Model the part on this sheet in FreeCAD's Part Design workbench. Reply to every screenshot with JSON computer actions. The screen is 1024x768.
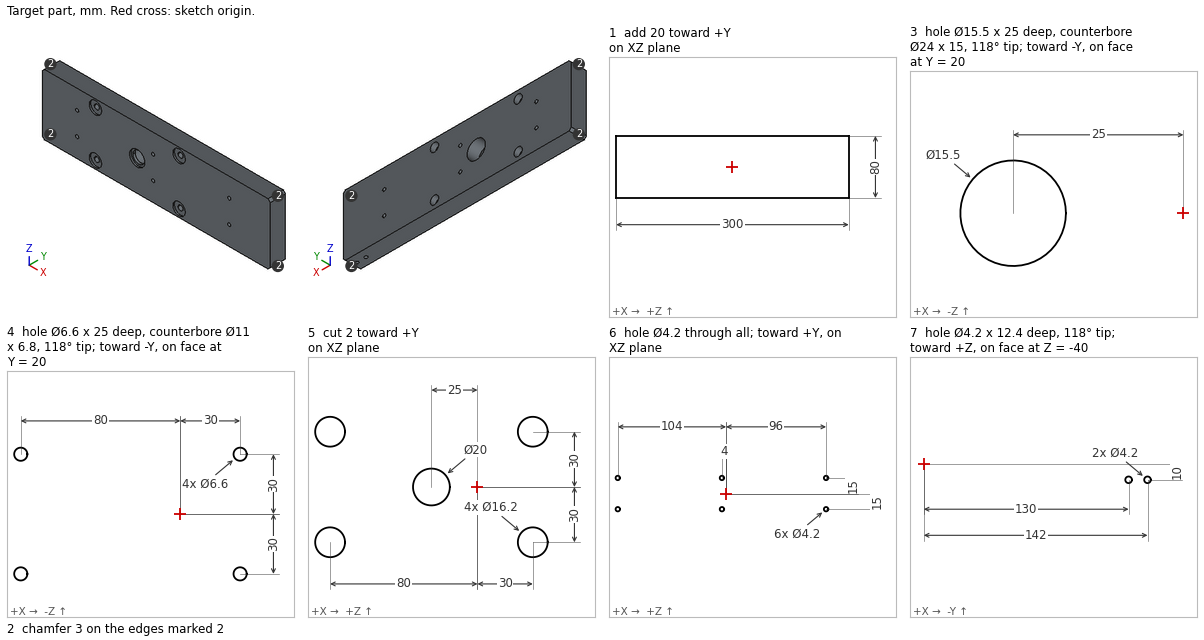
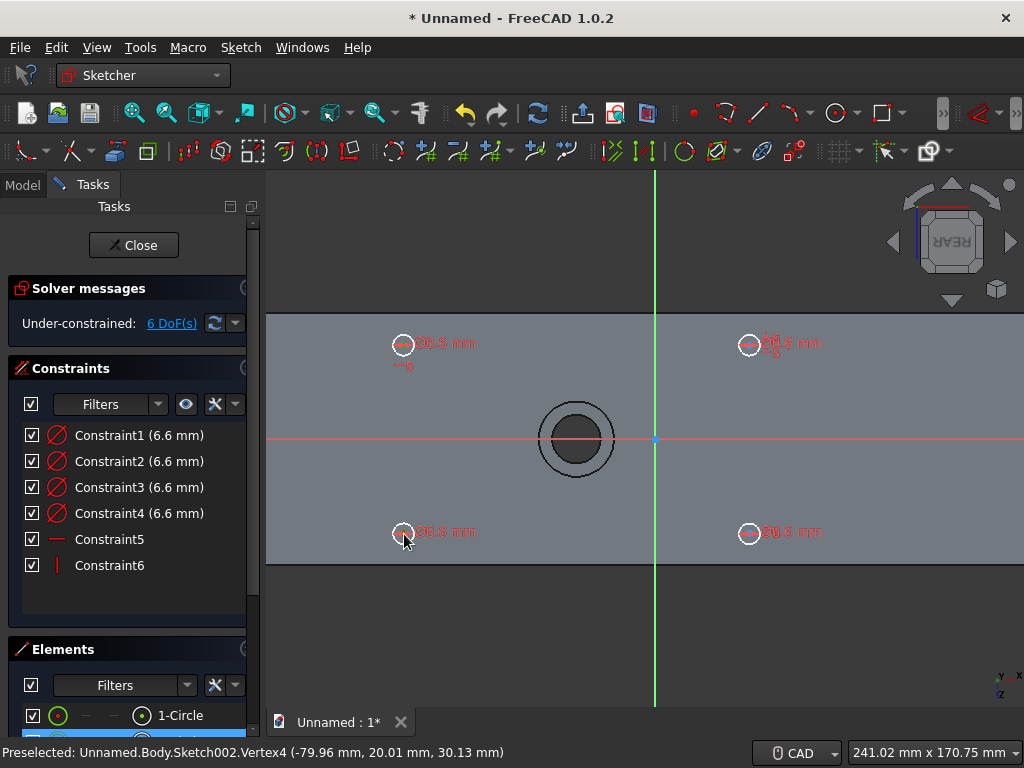
{"action": "key", "text": "v"}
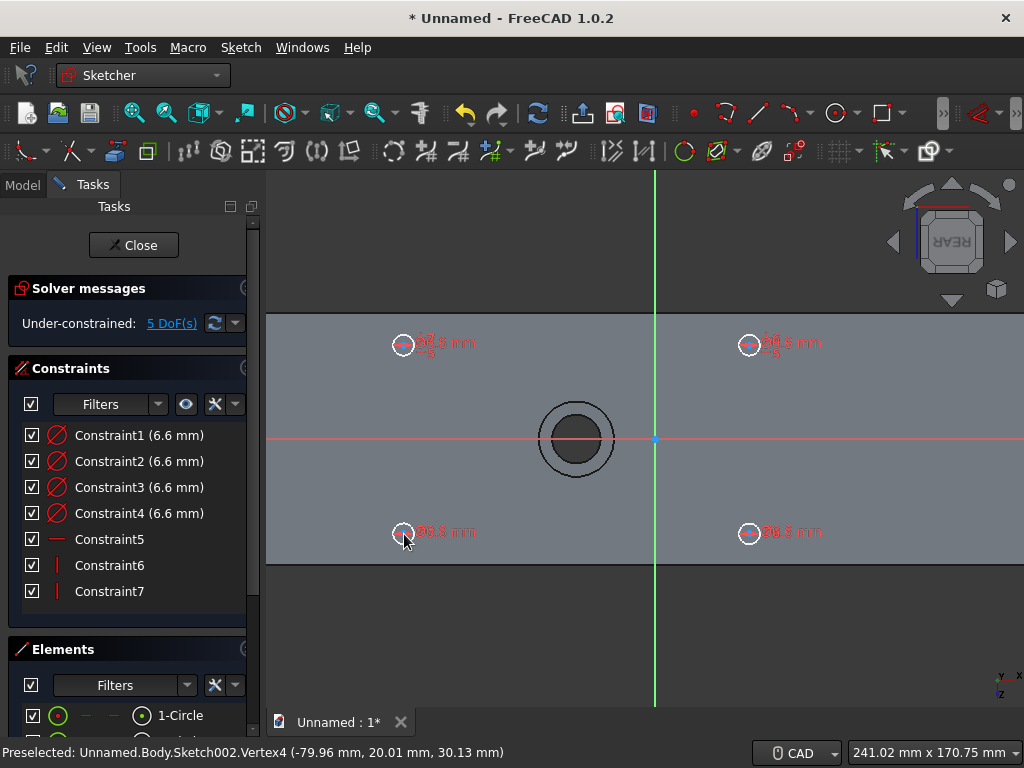
{"action": "left_click", "coordinate": [749, 534]}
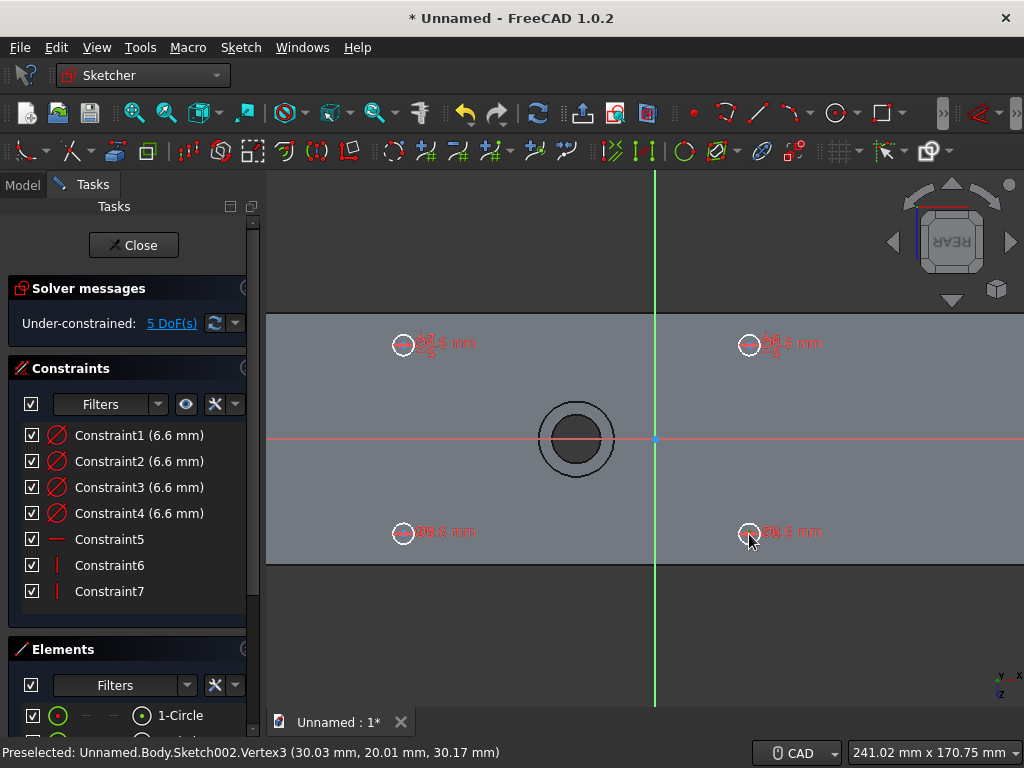
{"action": "left_click", "coordinate": [404, 534]}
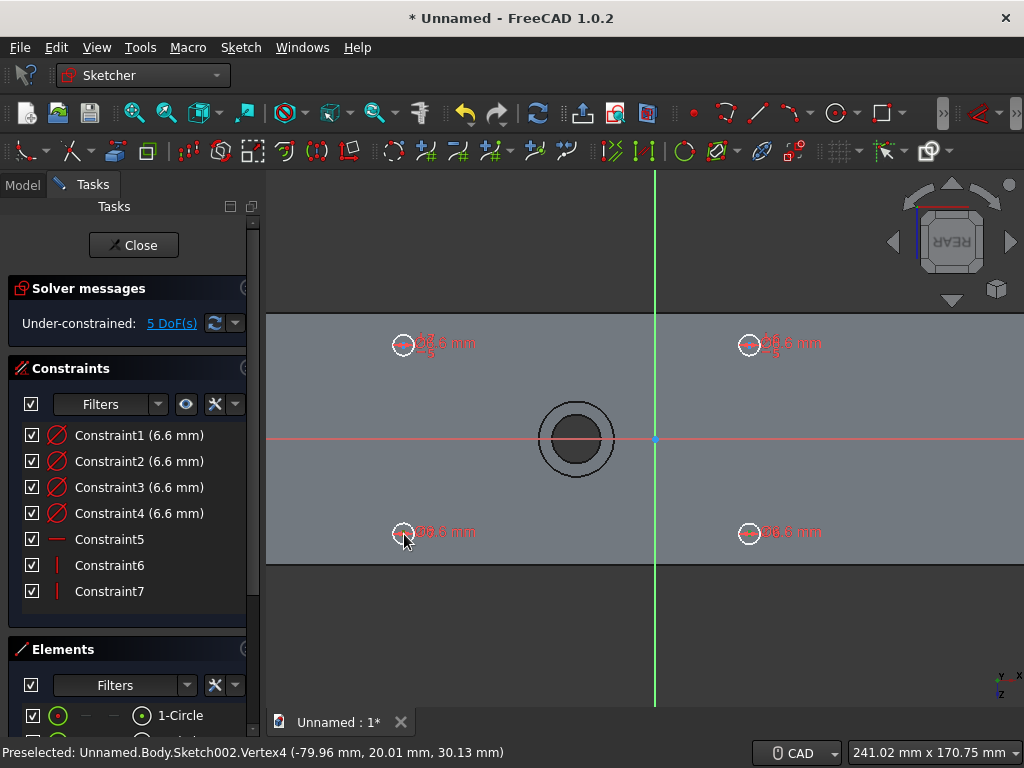
{"action": "key", "text": "h"}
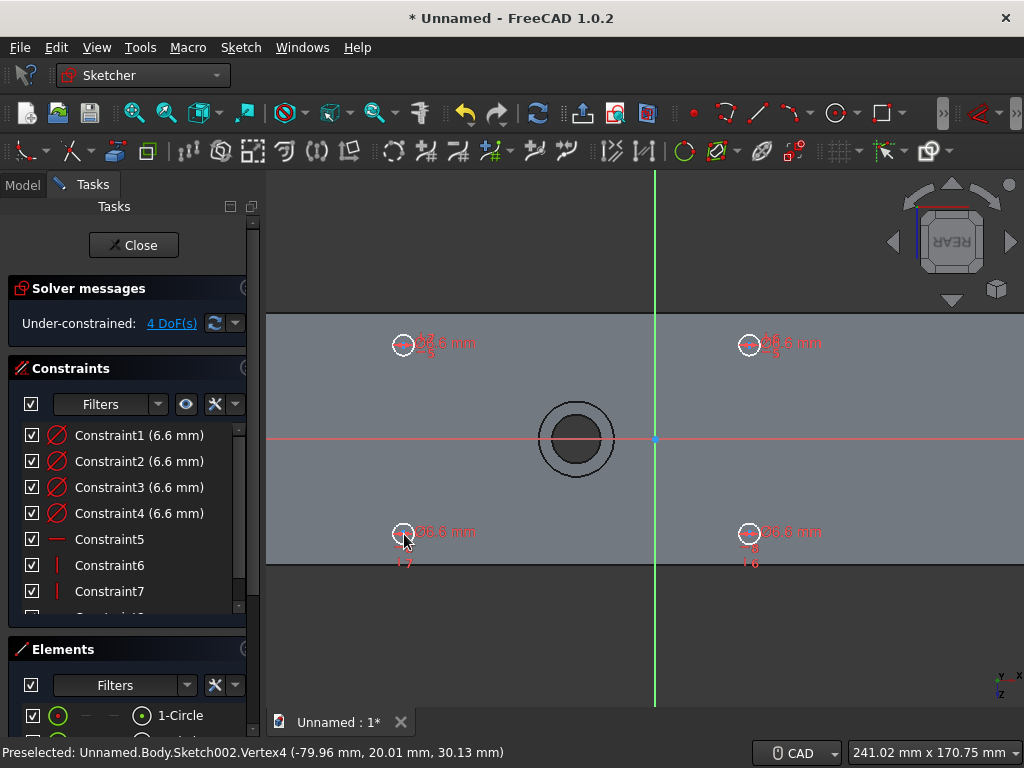
{"action": "left_click", "coordinate": [978, 114]}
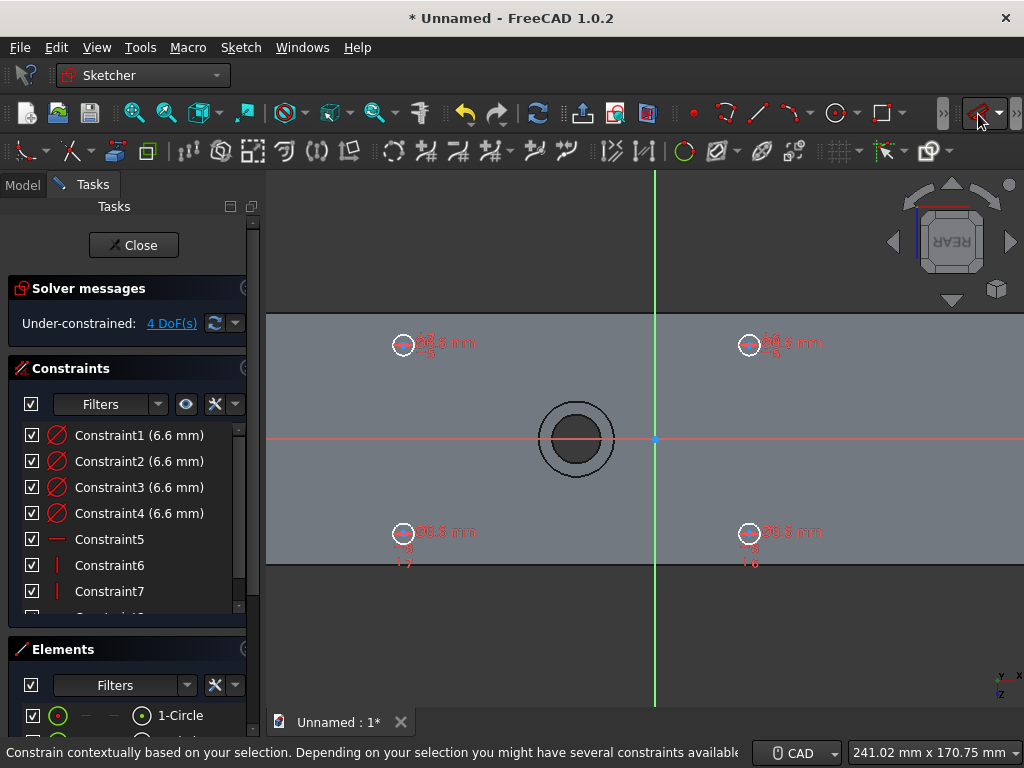
{"action": "left_click", "coordinate": [749, 345]}
{"action": "left_click", "coordinate": [702, 311]}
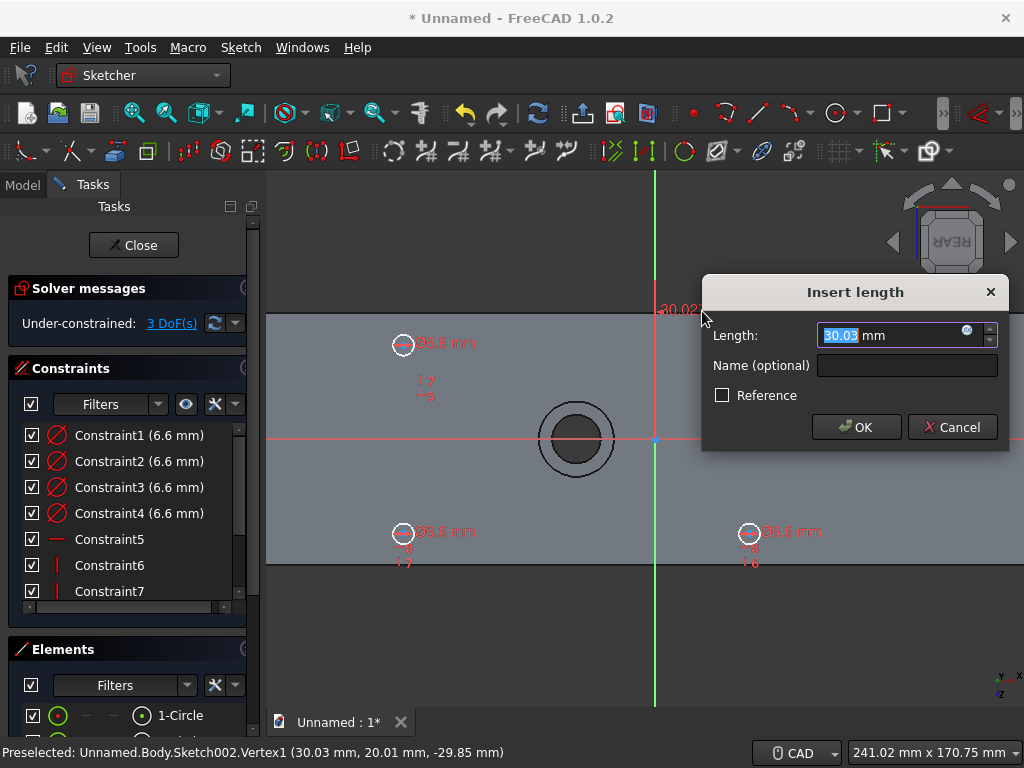
{"action": "type", "text": "30"}
{"action": "key", "text": "Return"}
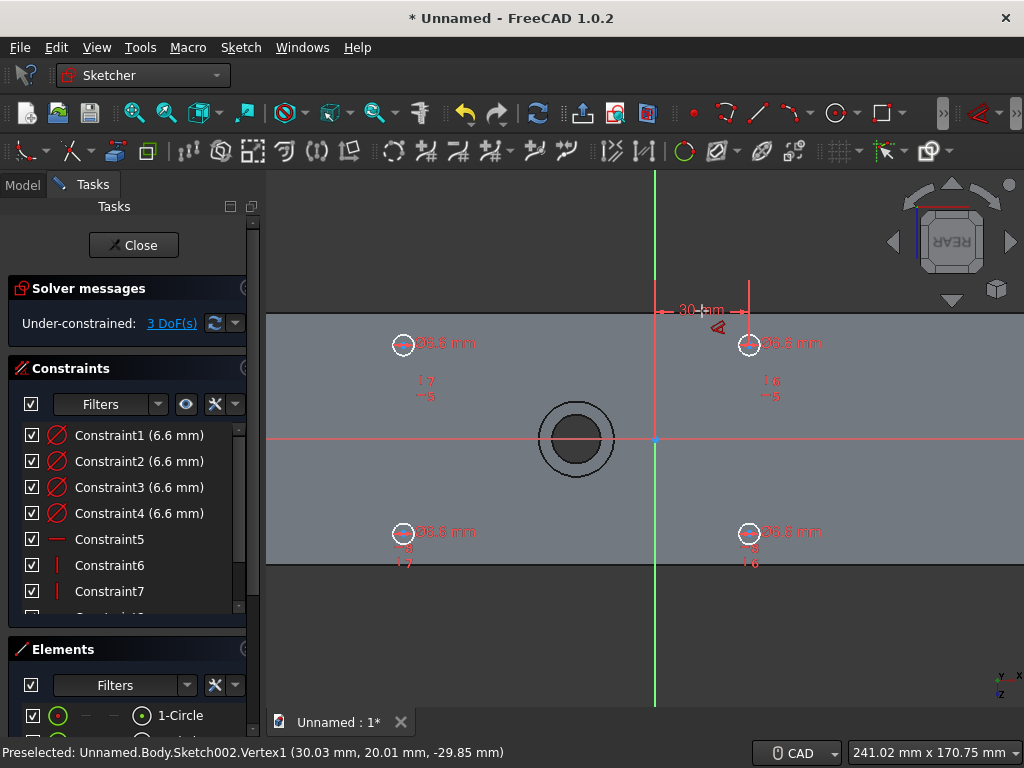
{"action": "left_click", "coordinate": [749, 345]}
{"action": "left_click", "coordinate": [783, 392]}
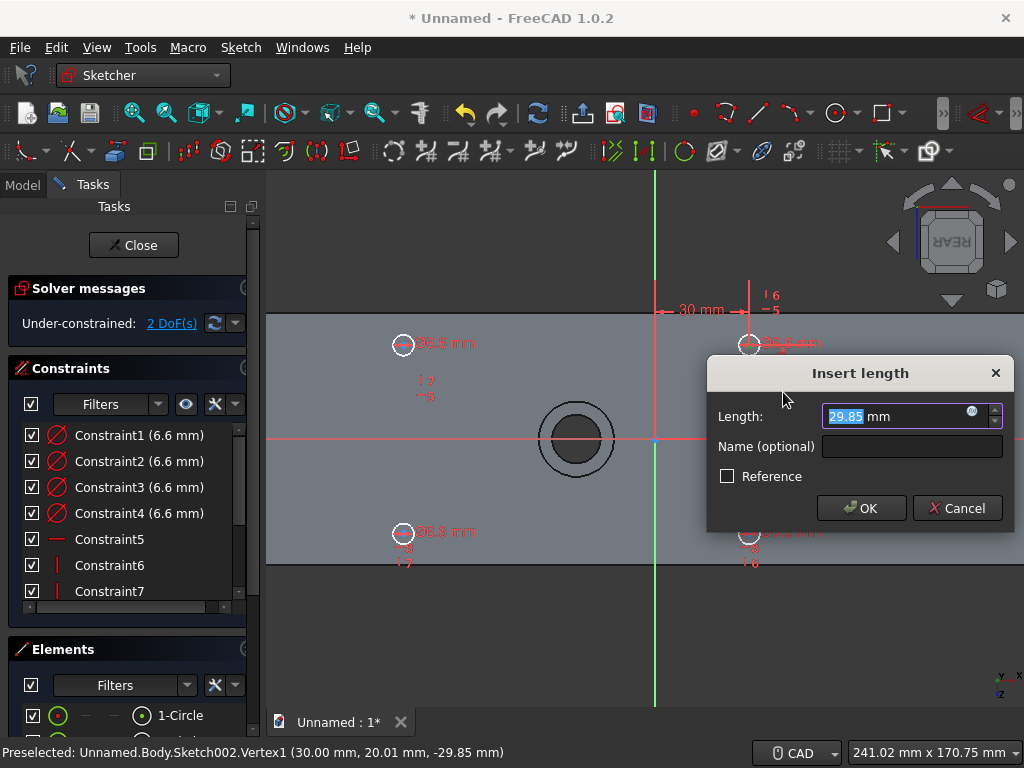
{"action": "type", "text": "30"}
{"action": "key", "text": "Return"}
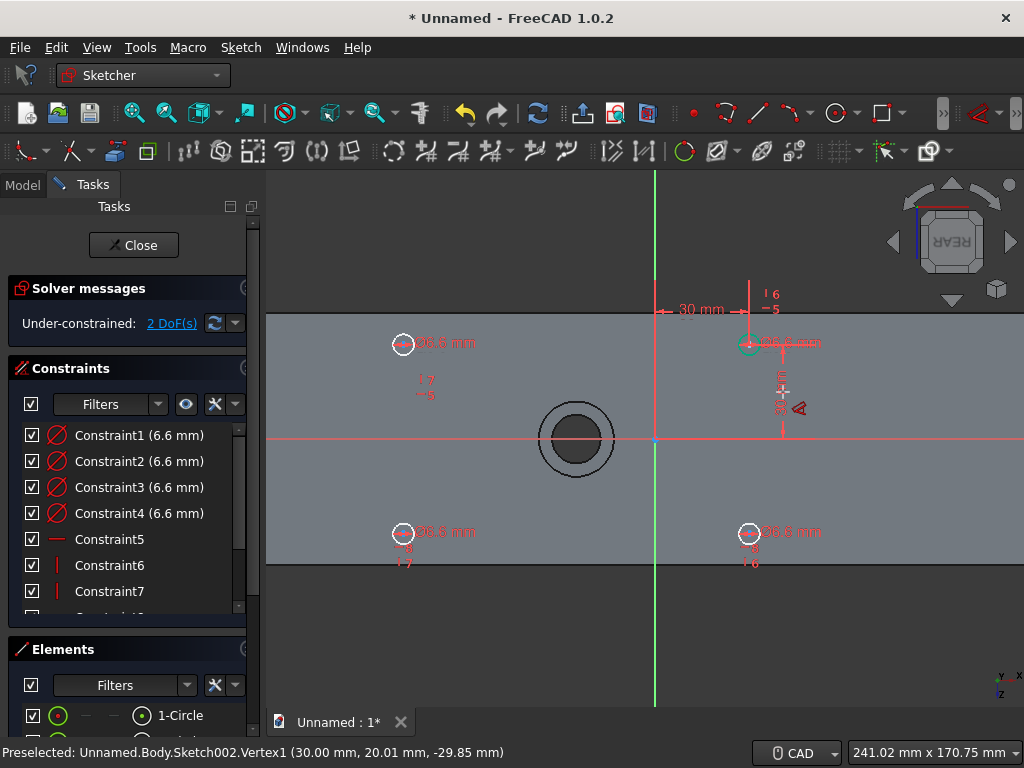
{"action": "left_click", "coordinate": [404, 345]}
{"action": "left_click", "coordinate": [529, 311]}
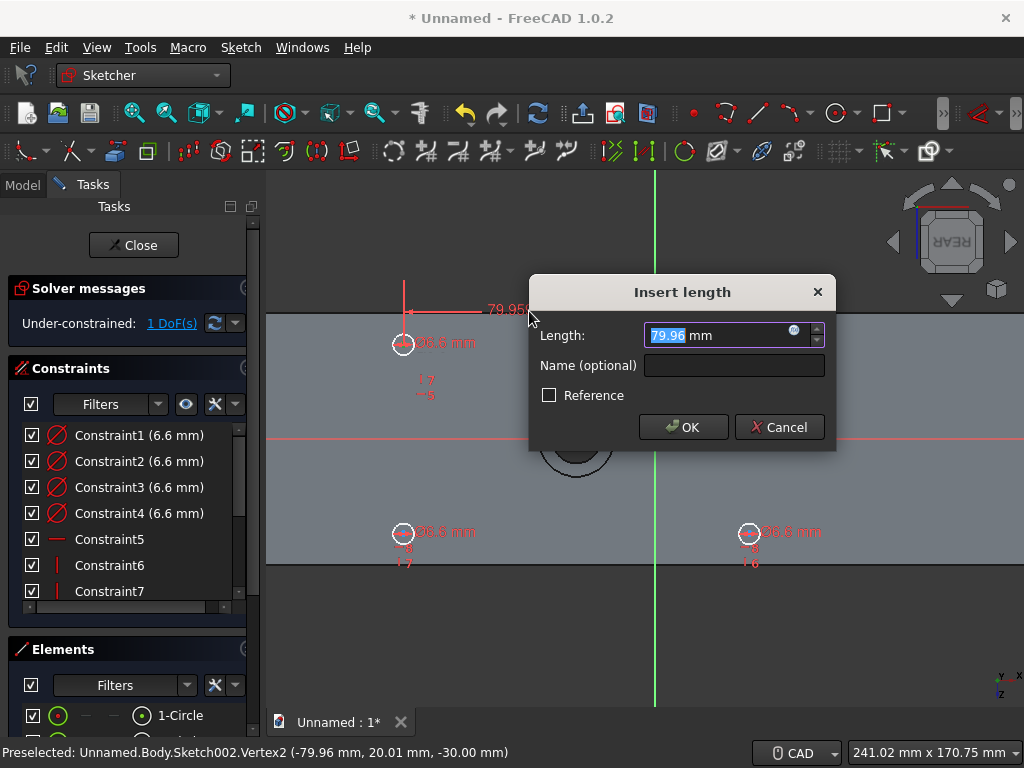
{"action": "type", "text": "80"}
{"action": "key", "text": "Return"}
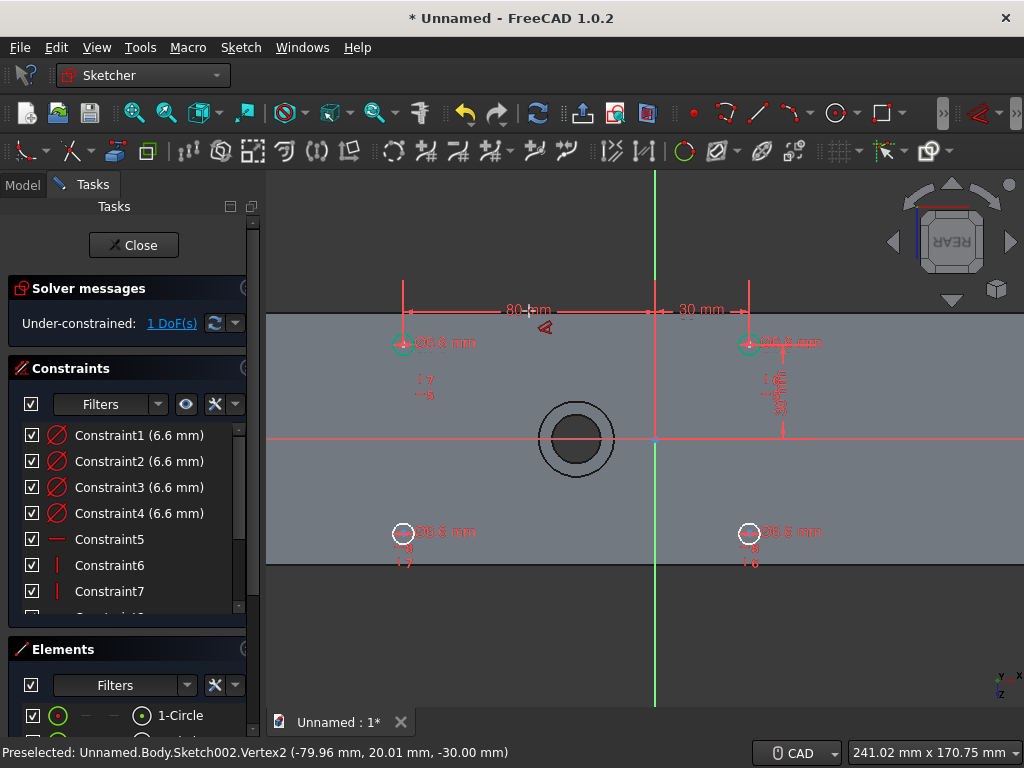
{"action": "left_click", "coordinate": [749, 534]}
{"action": "left_click", "coordinate": [783, 486]}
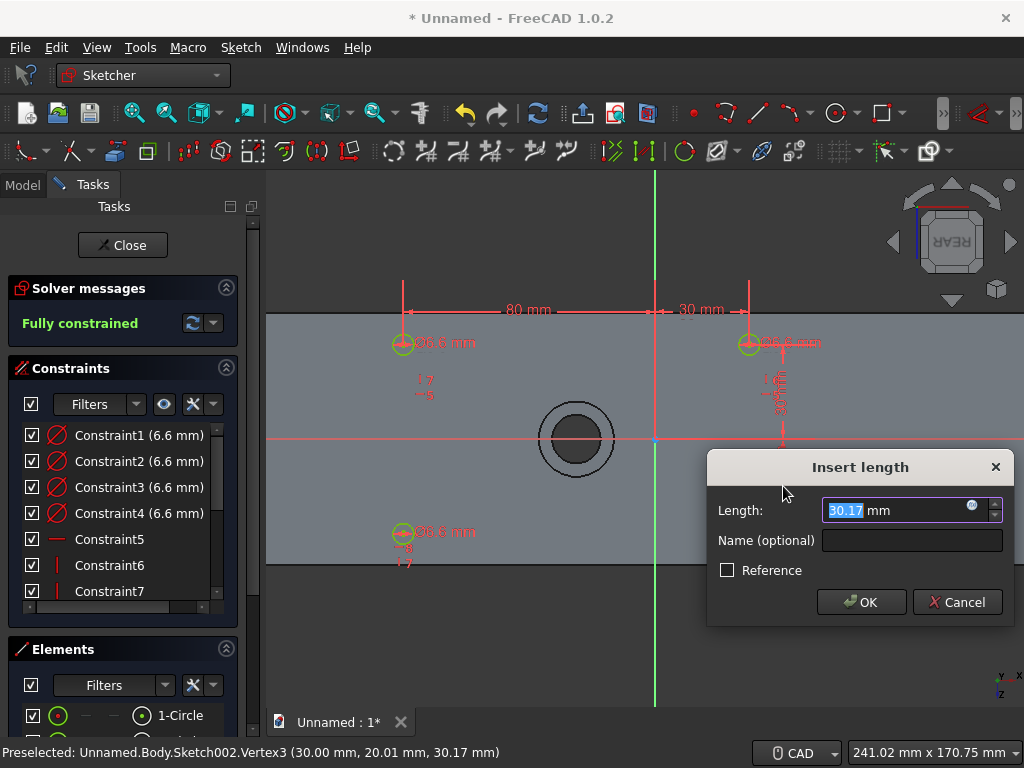
{"action": "type", "text": "30"}
{"action": "key", "text": "Return"}
{"action": "key", "text": "Escape"}